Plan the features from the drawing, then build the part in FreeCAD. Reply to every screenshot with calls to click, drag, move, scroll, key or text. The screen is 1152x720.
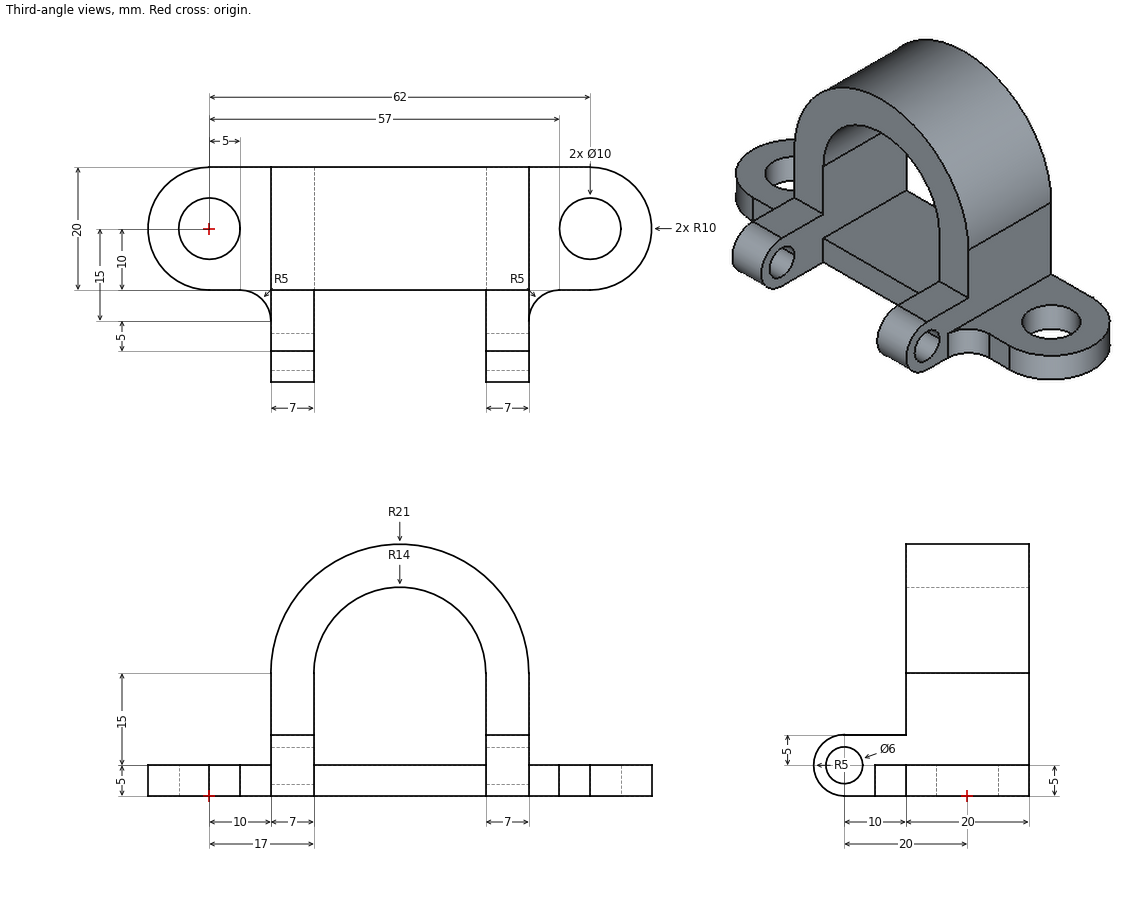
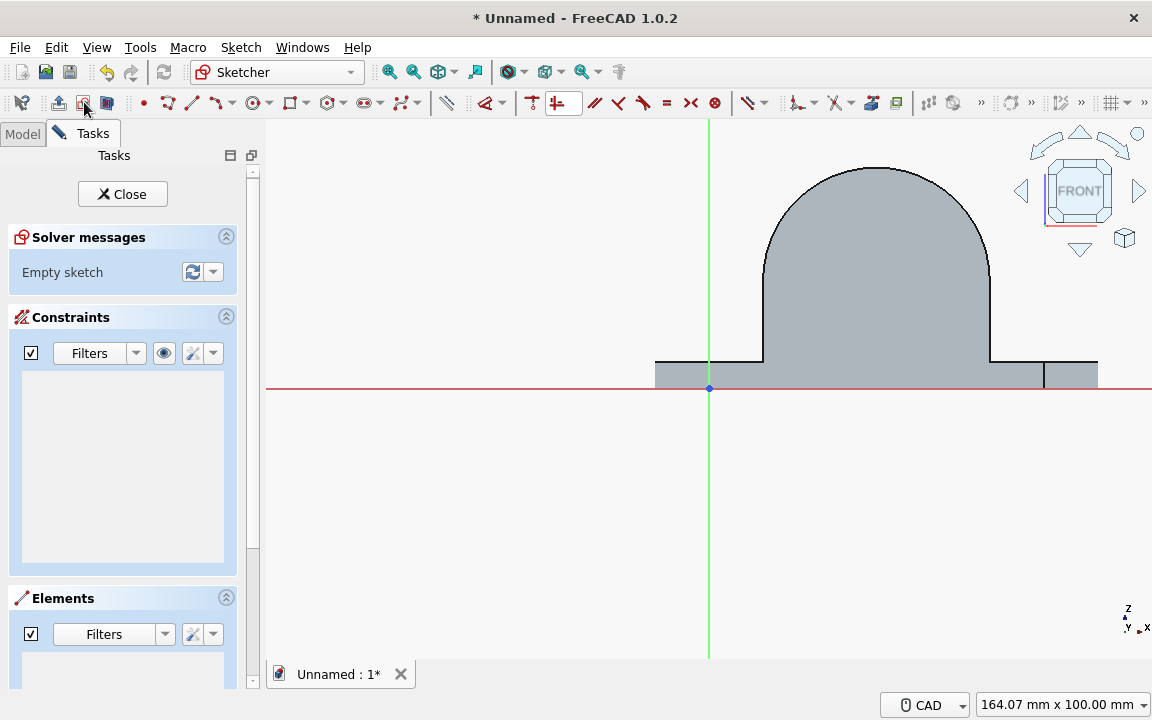
scroll(987, 186, up, 3)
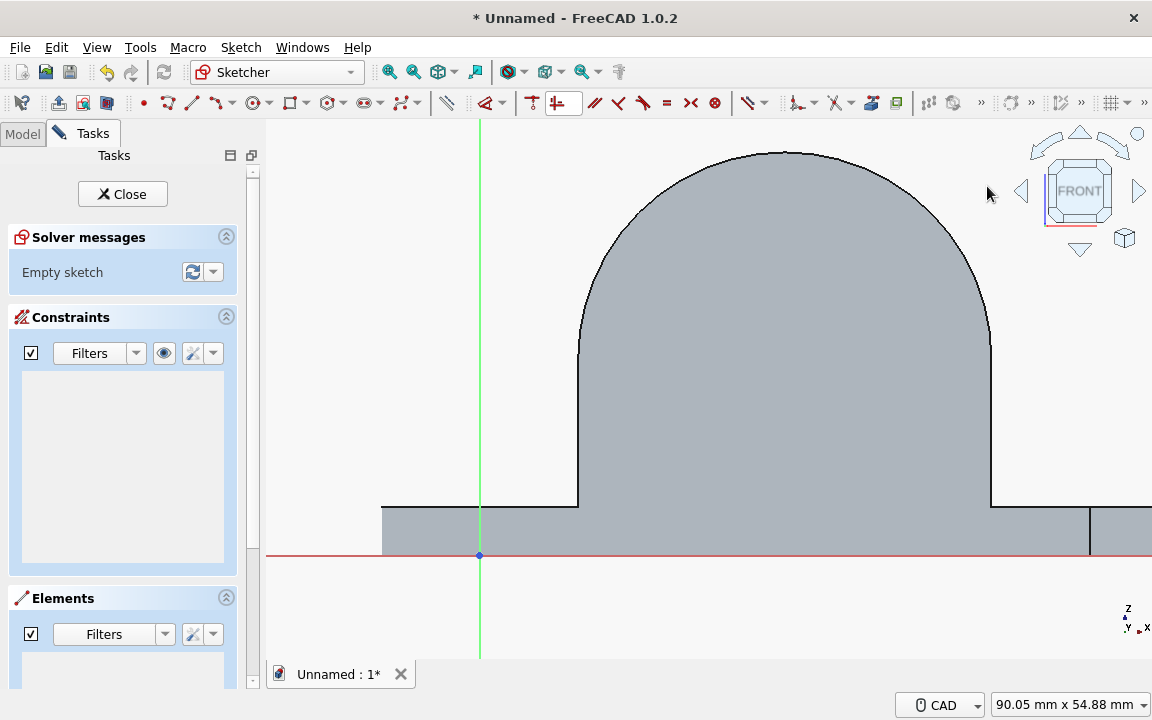
key(g)
key(m)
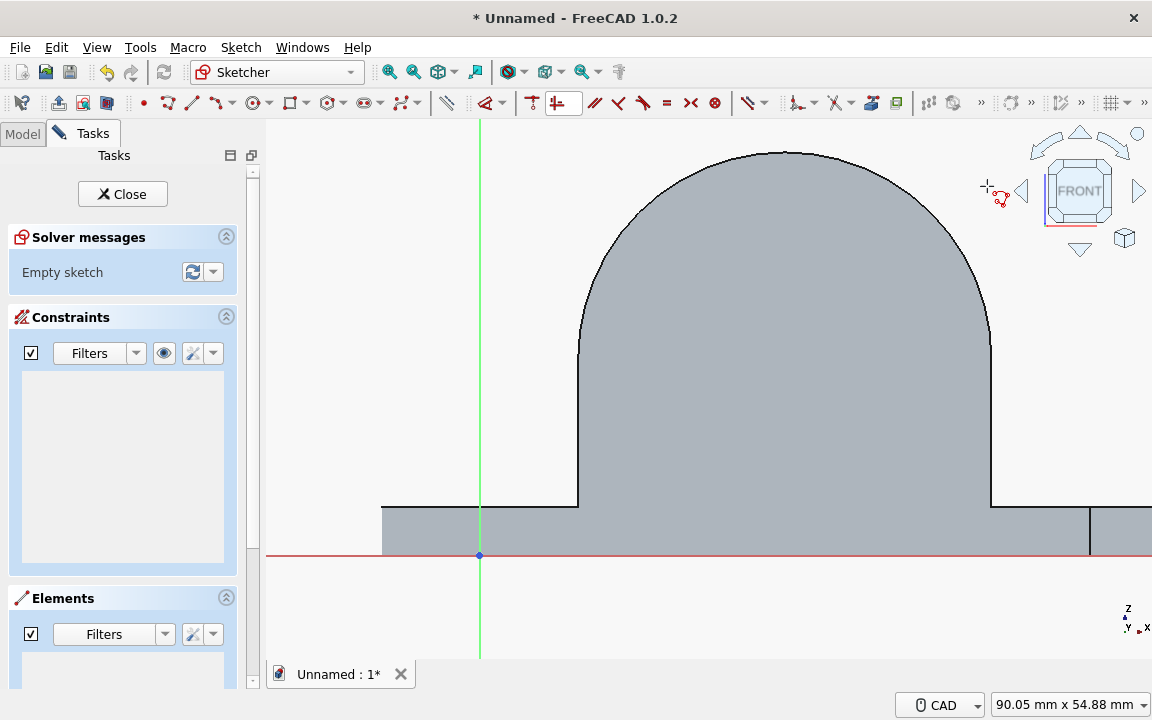
click(647, 359)
click(647, 507)
click(923, 507)
click(923, 359)
right_click(923, 359)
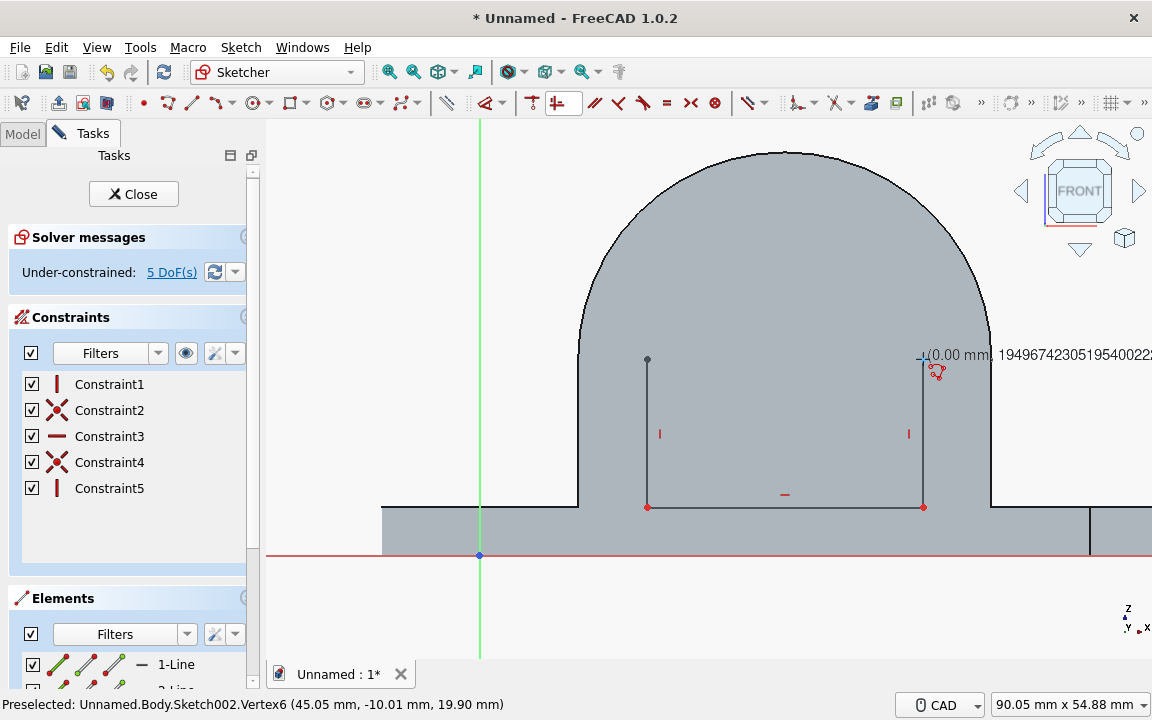
click(216, 104)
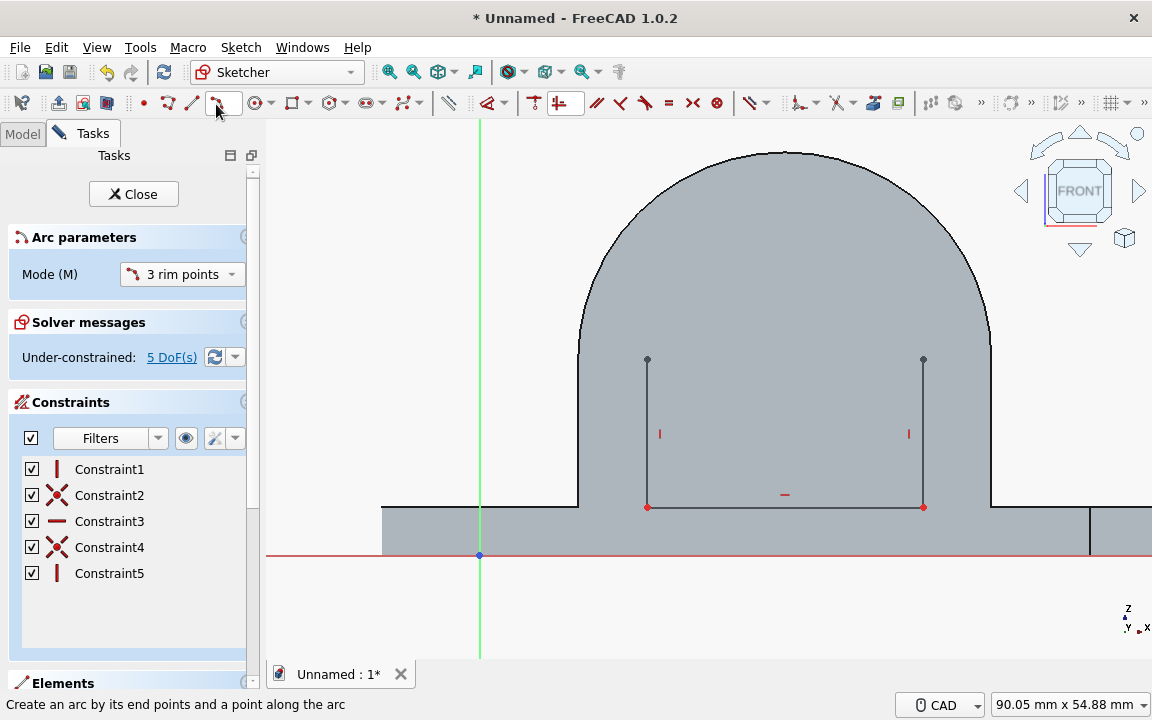
click(923, 360)
click(647, 360)
click(785, 221)
key(Escape)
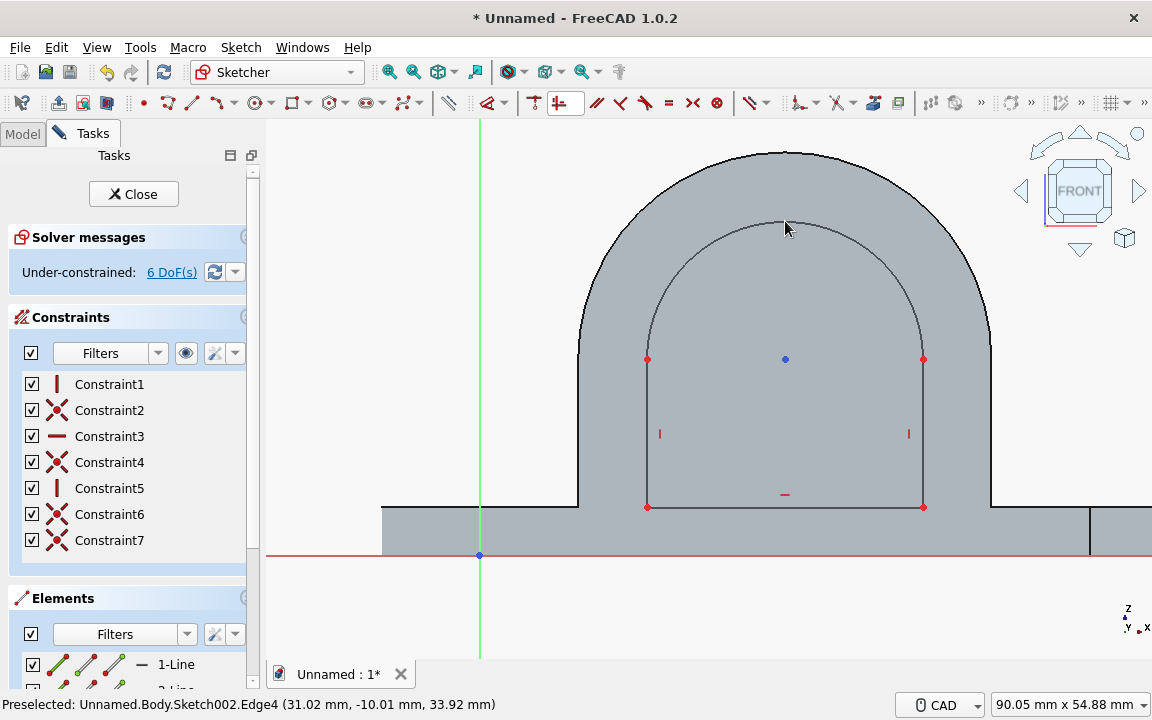
click(647, 404)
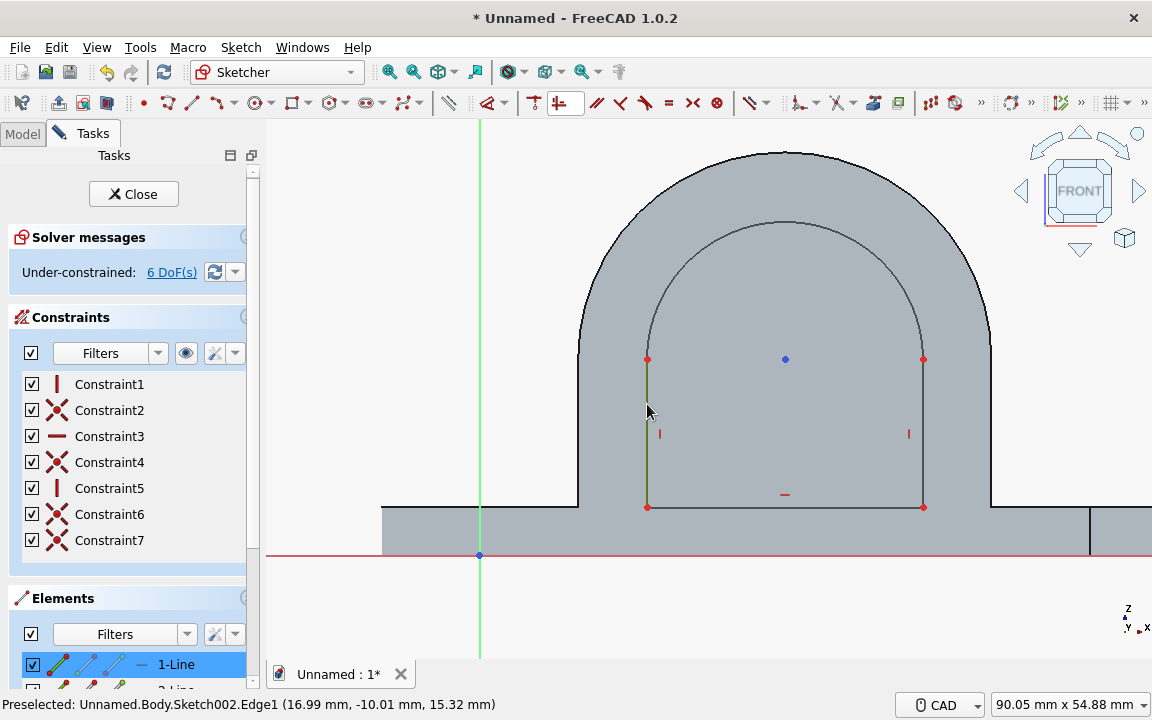
click(866, 248)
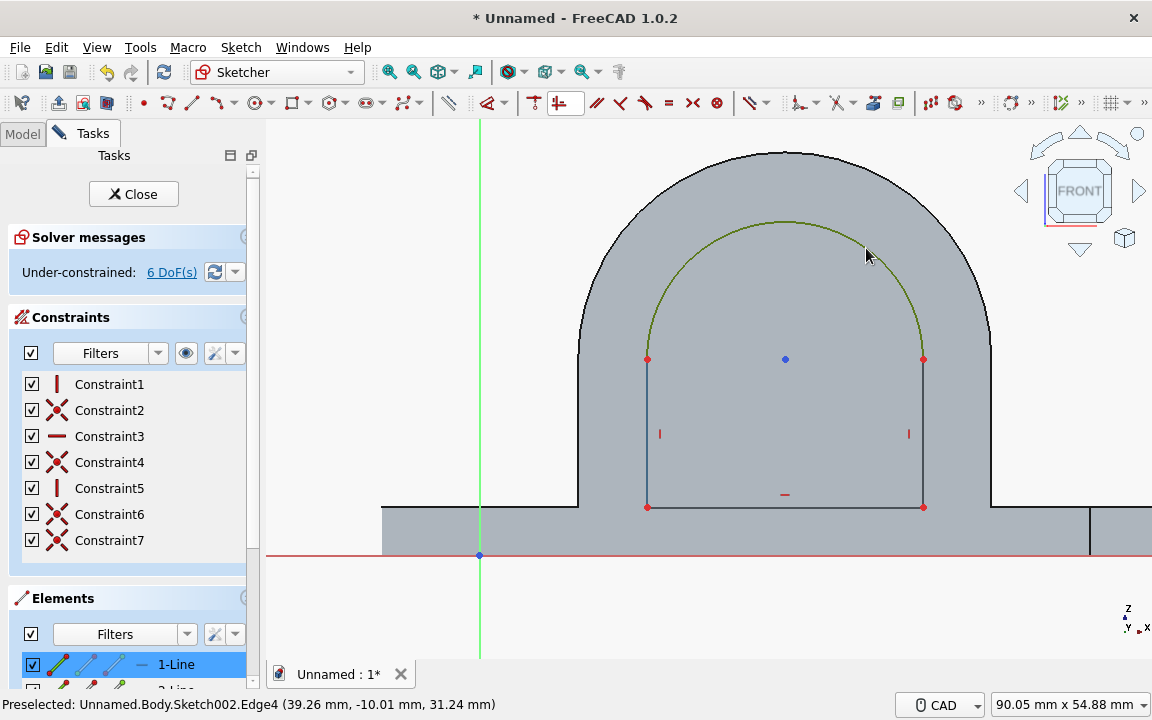
click(646, 104)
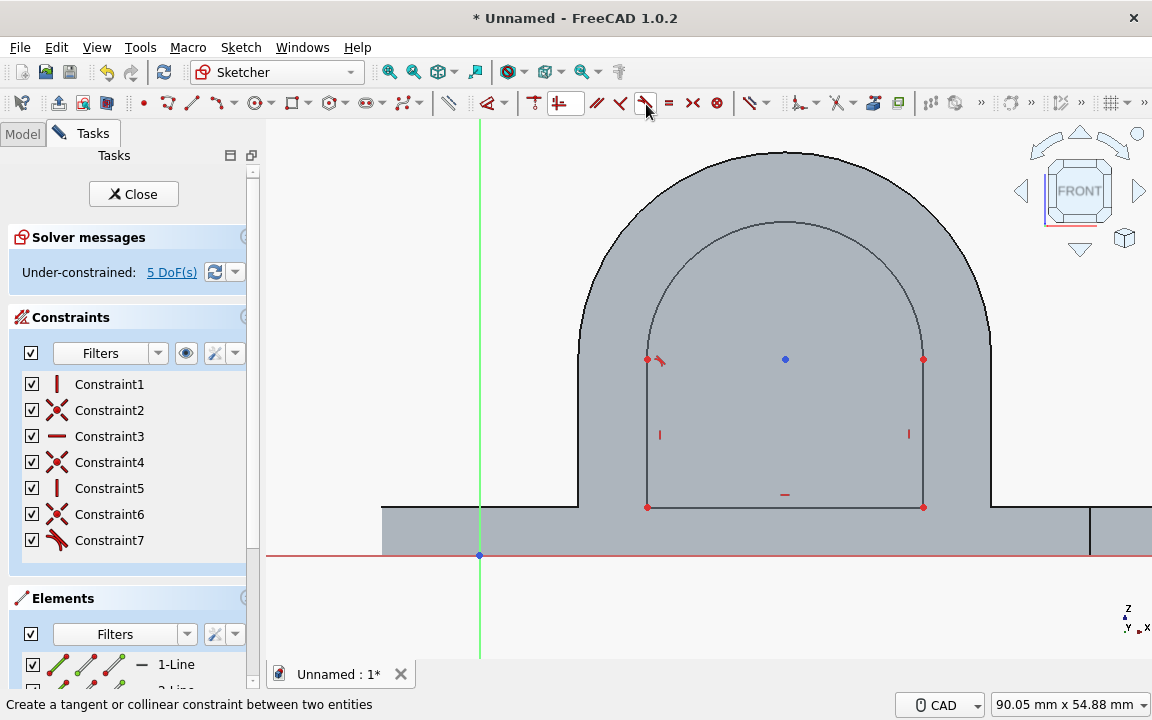
click(923, 464)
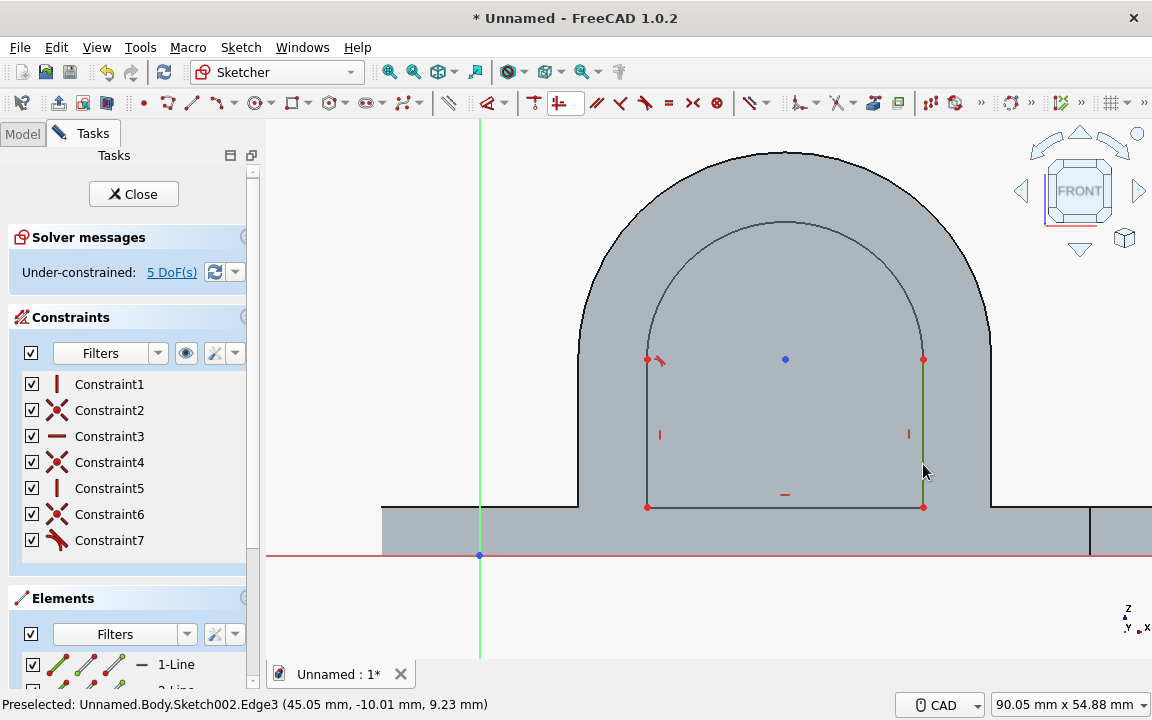
click(866, 248)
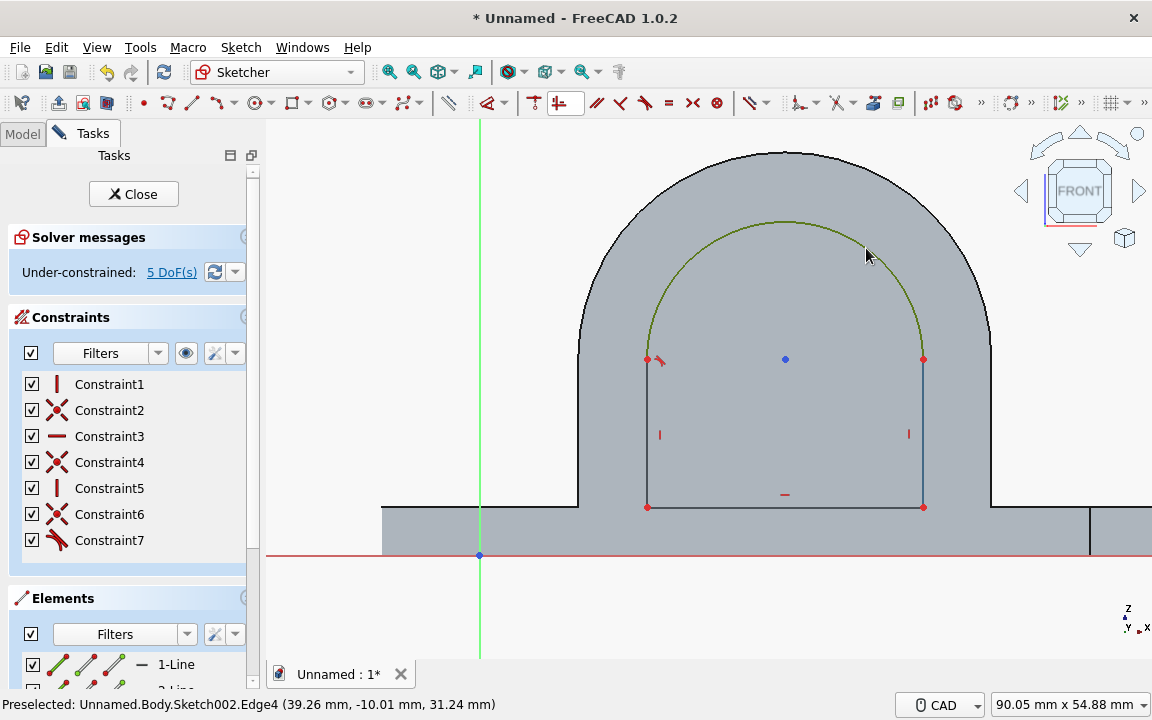
click(646, 104)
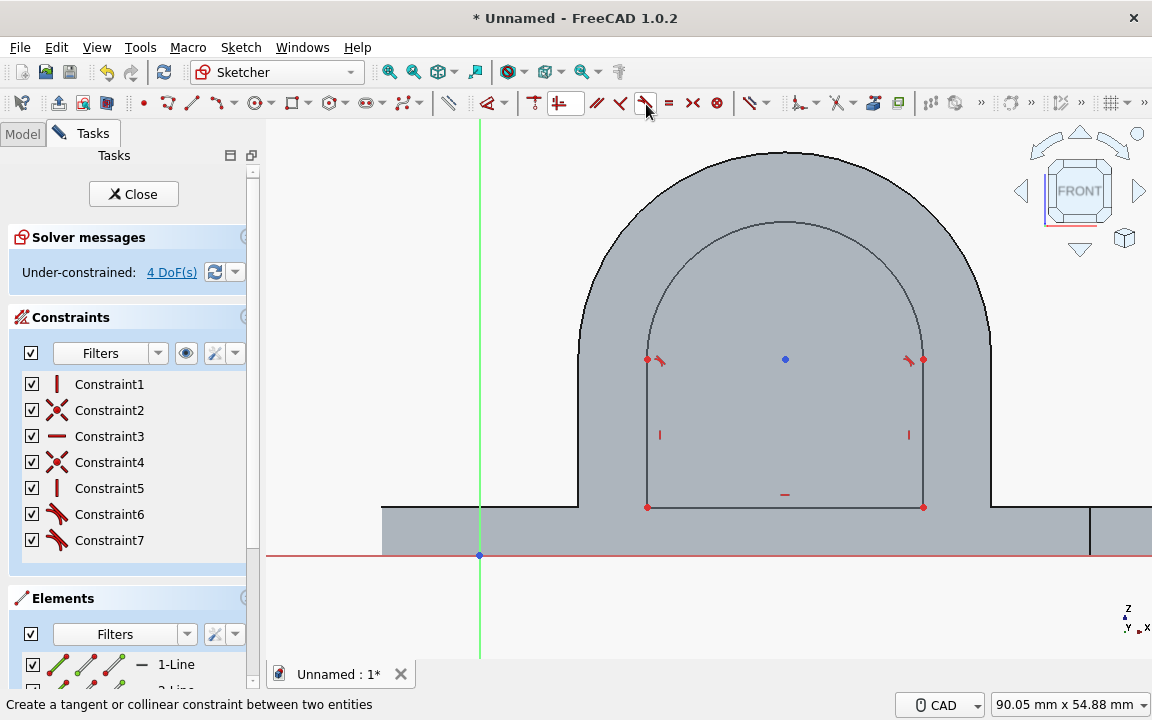
click(488, 104)